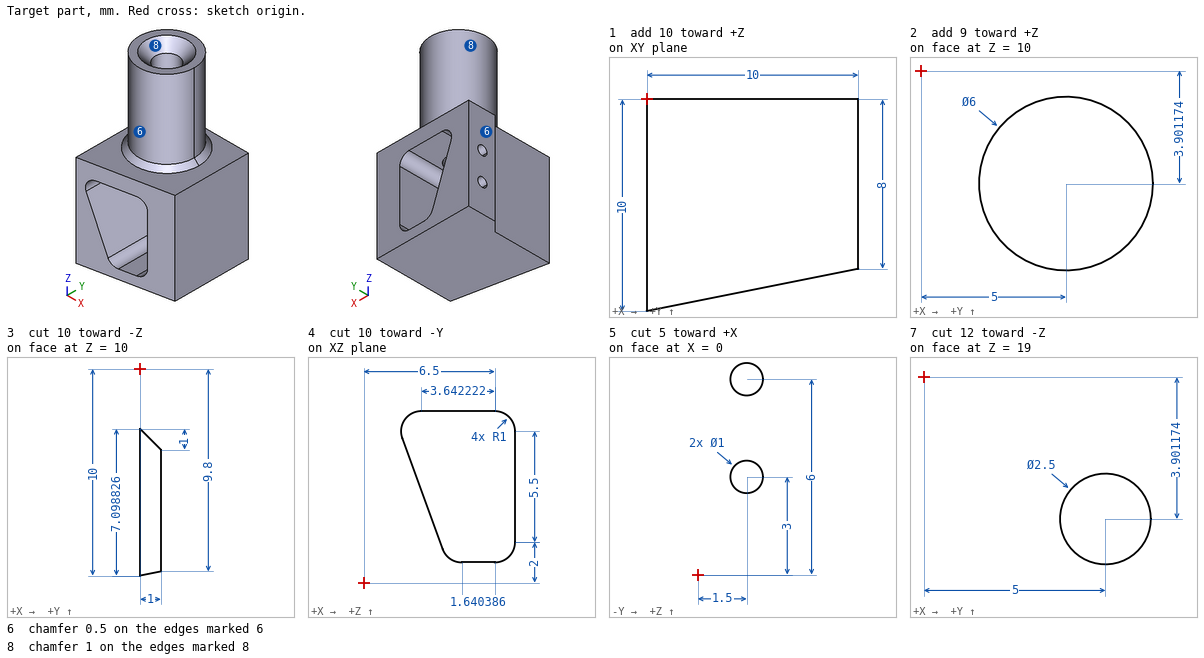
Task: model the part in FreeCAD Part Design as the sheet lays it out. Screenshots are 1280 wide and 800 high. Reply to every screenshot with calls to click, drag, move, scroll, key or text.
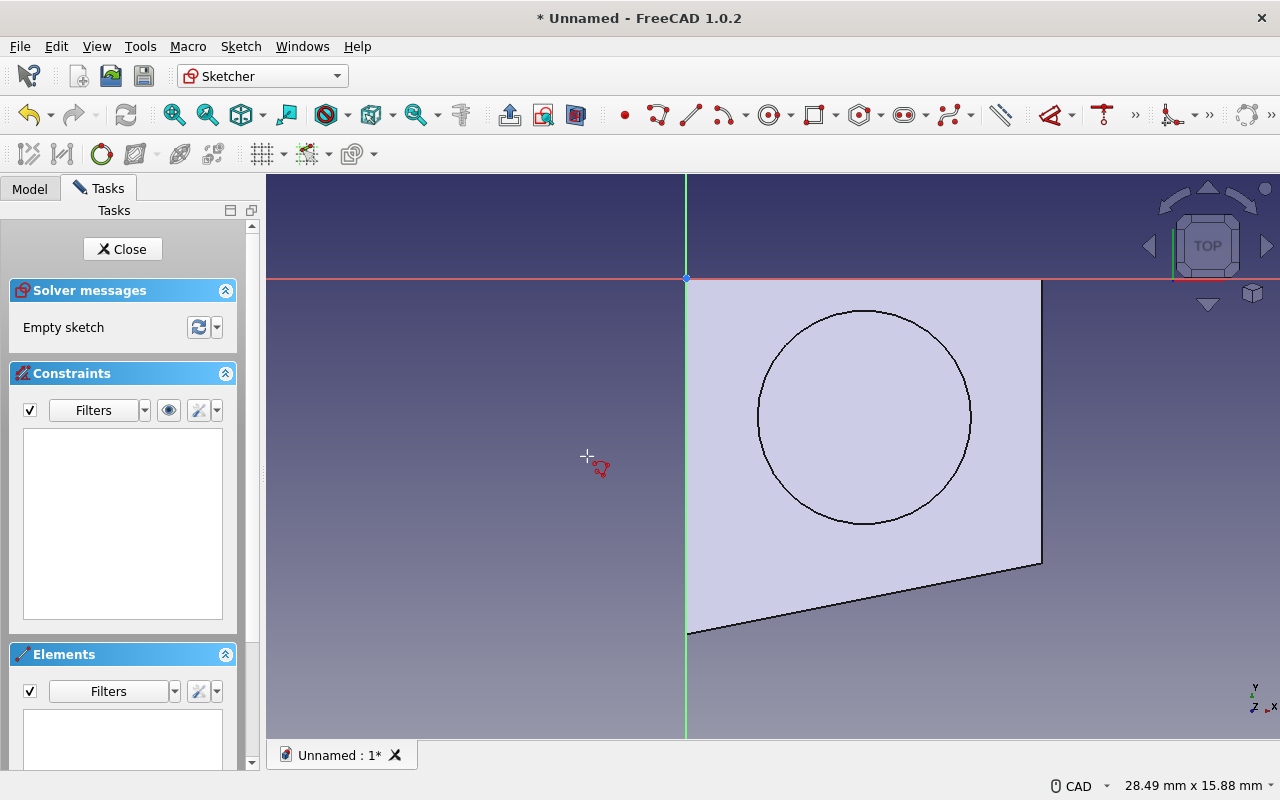
click(686, 382)
click(695, 634)
click(722, 627)
click(722, 417)
click(686, 383)
key(Escape)
key(Escape)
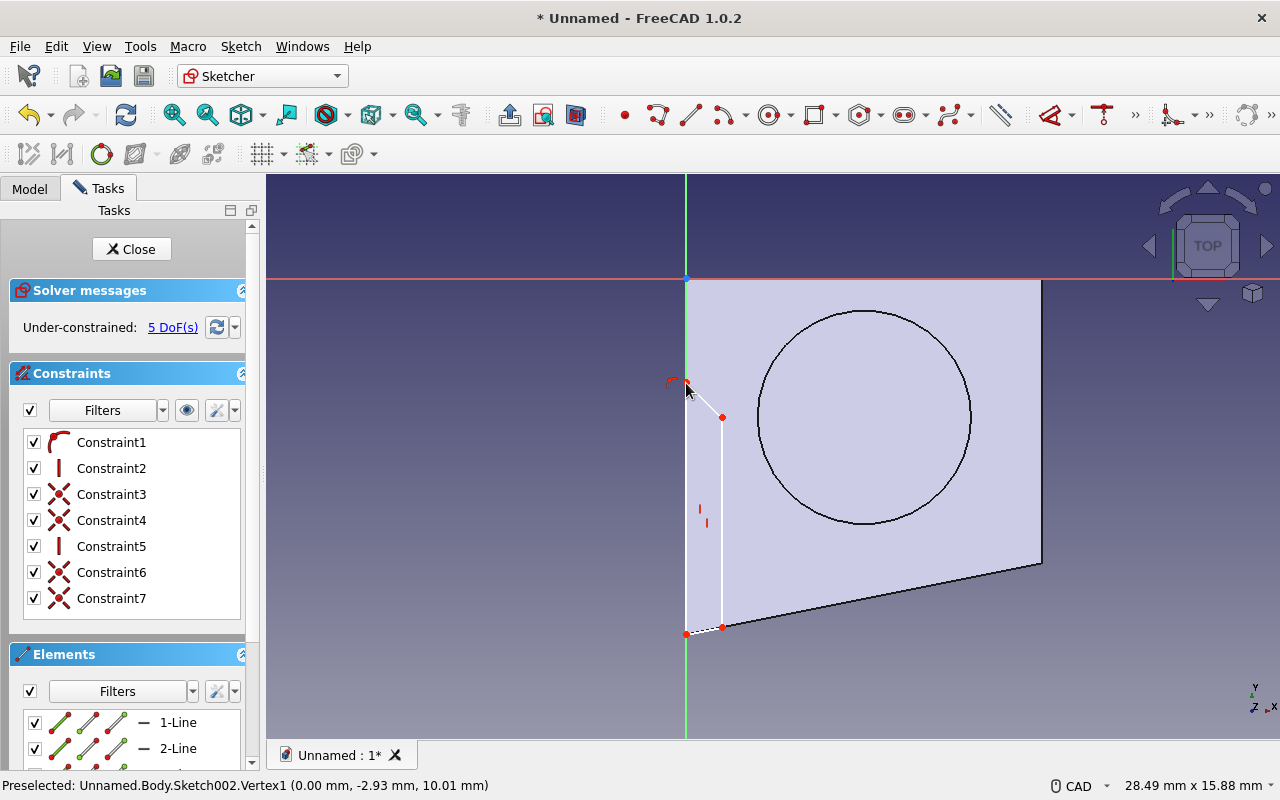
key(d)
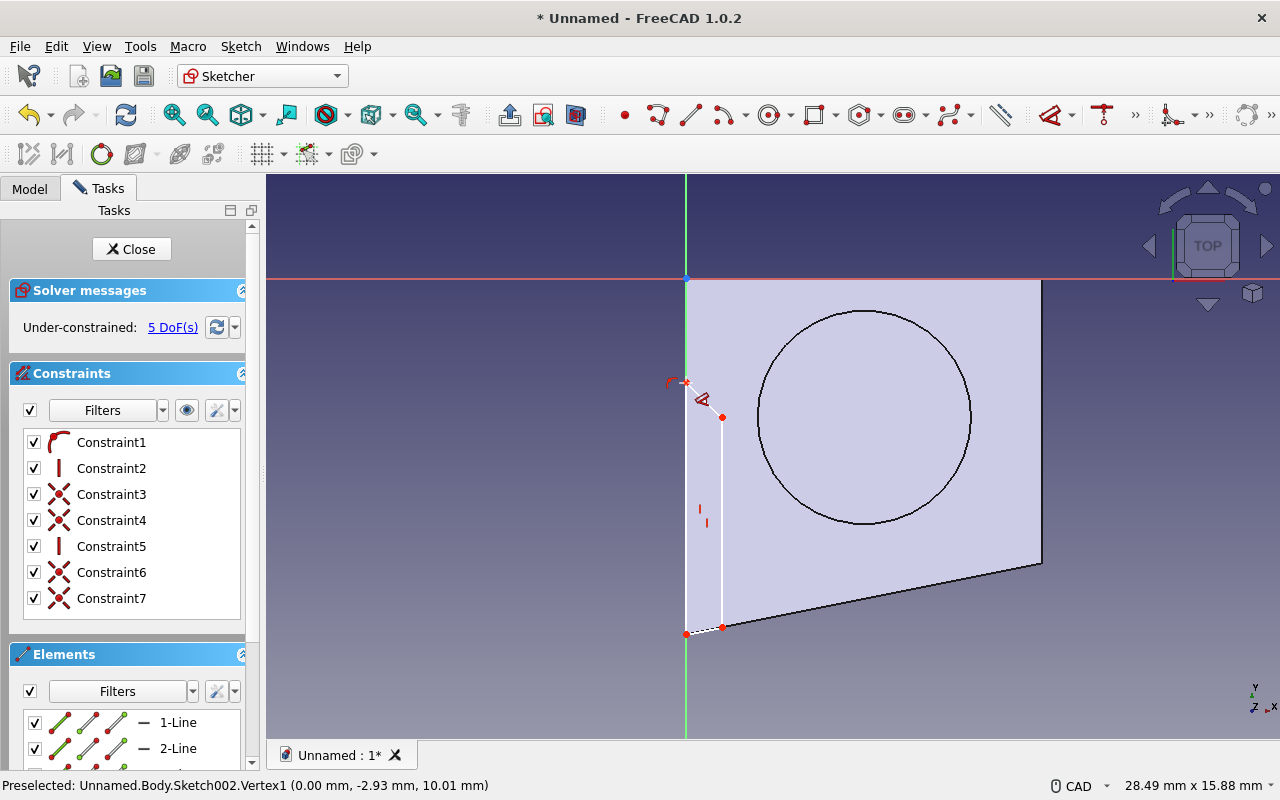
click(722, 628)
click(704, 245)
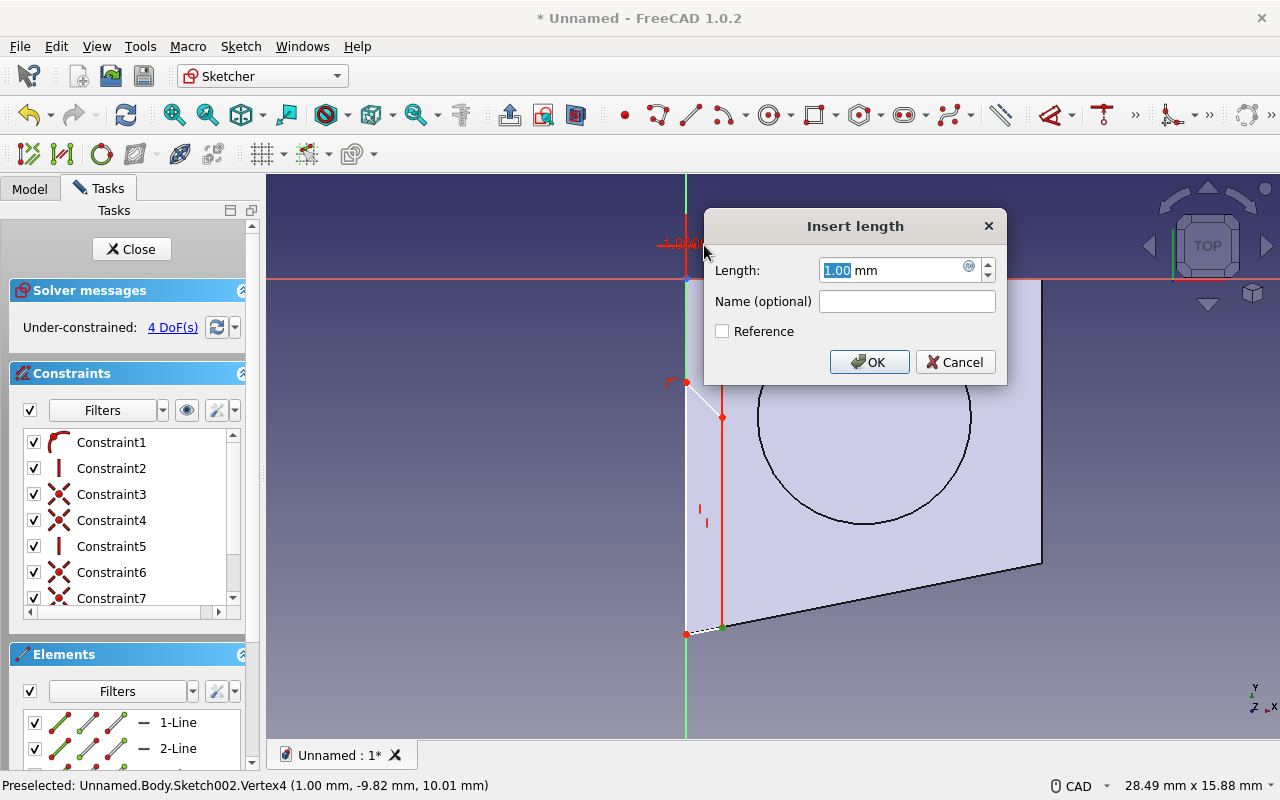
text(1)
key(Return)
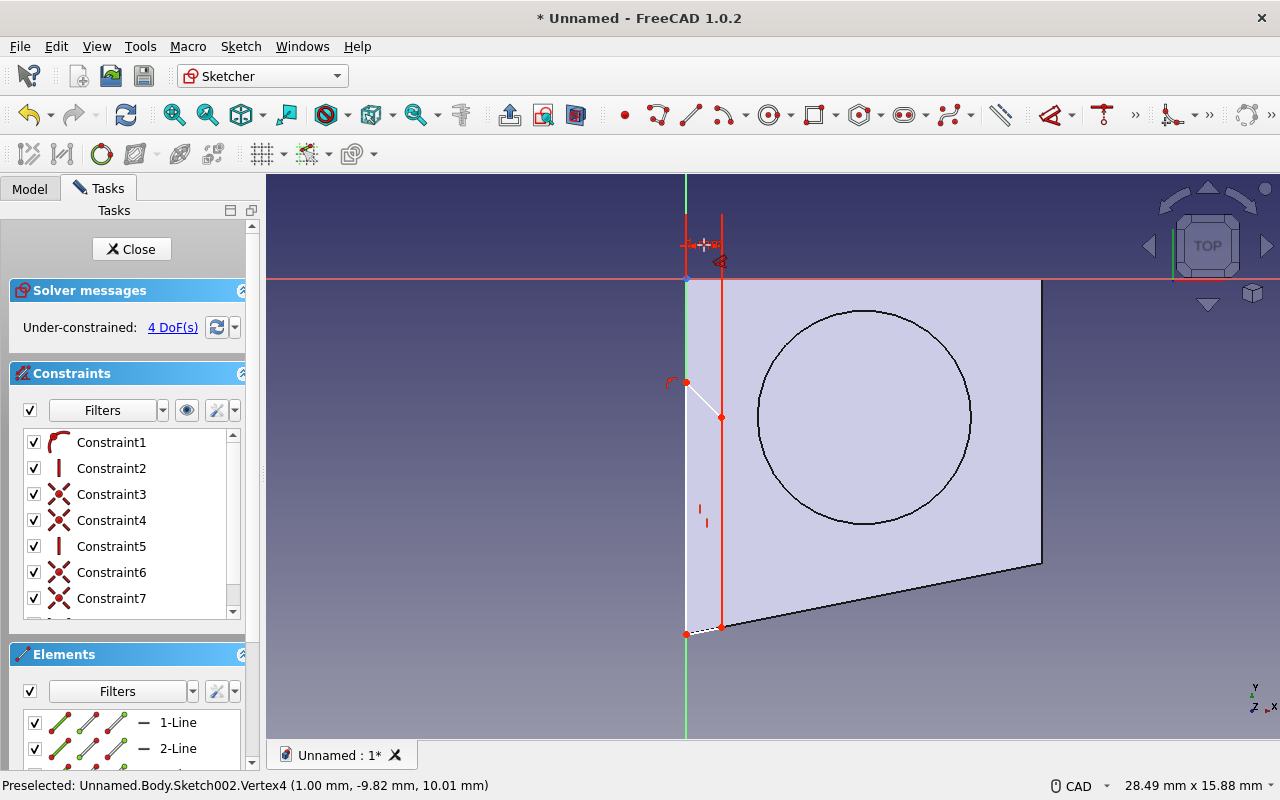
click(711, 408)
click(756, 401)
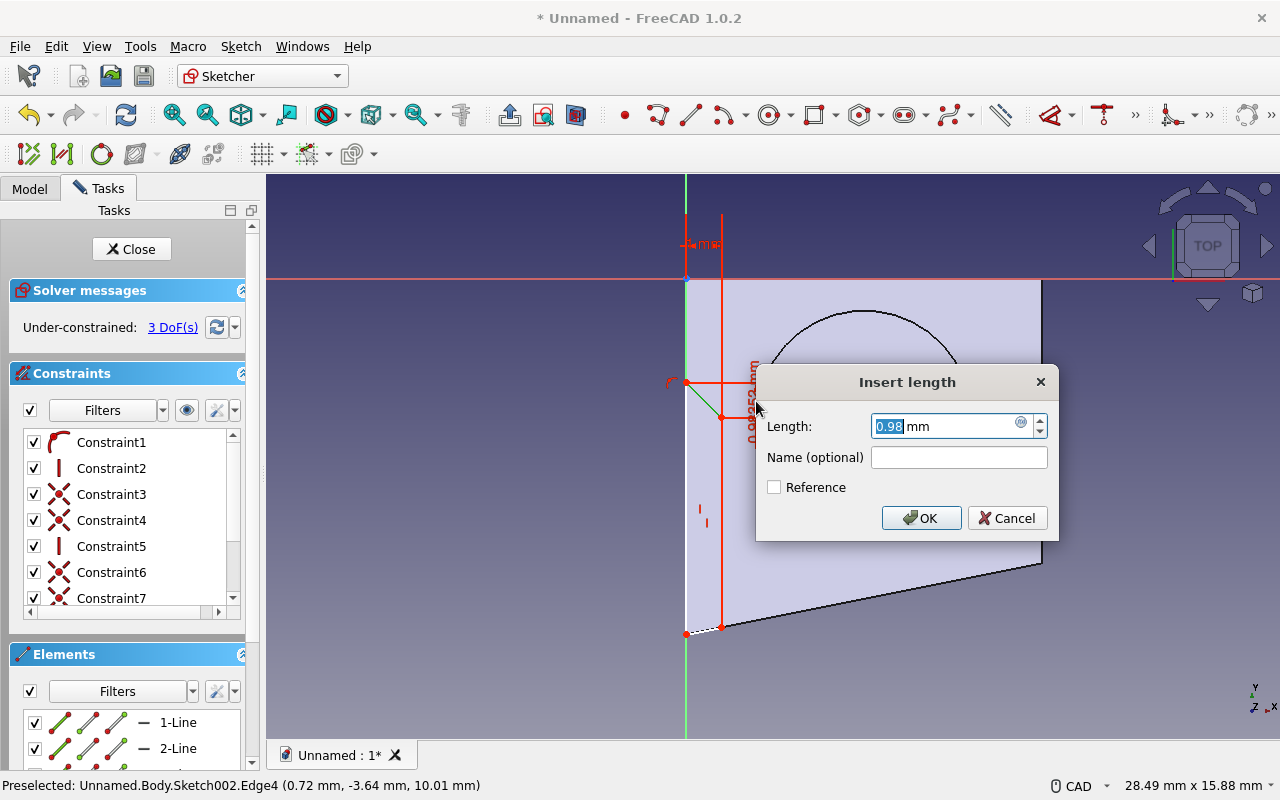
text(1)
key(Return)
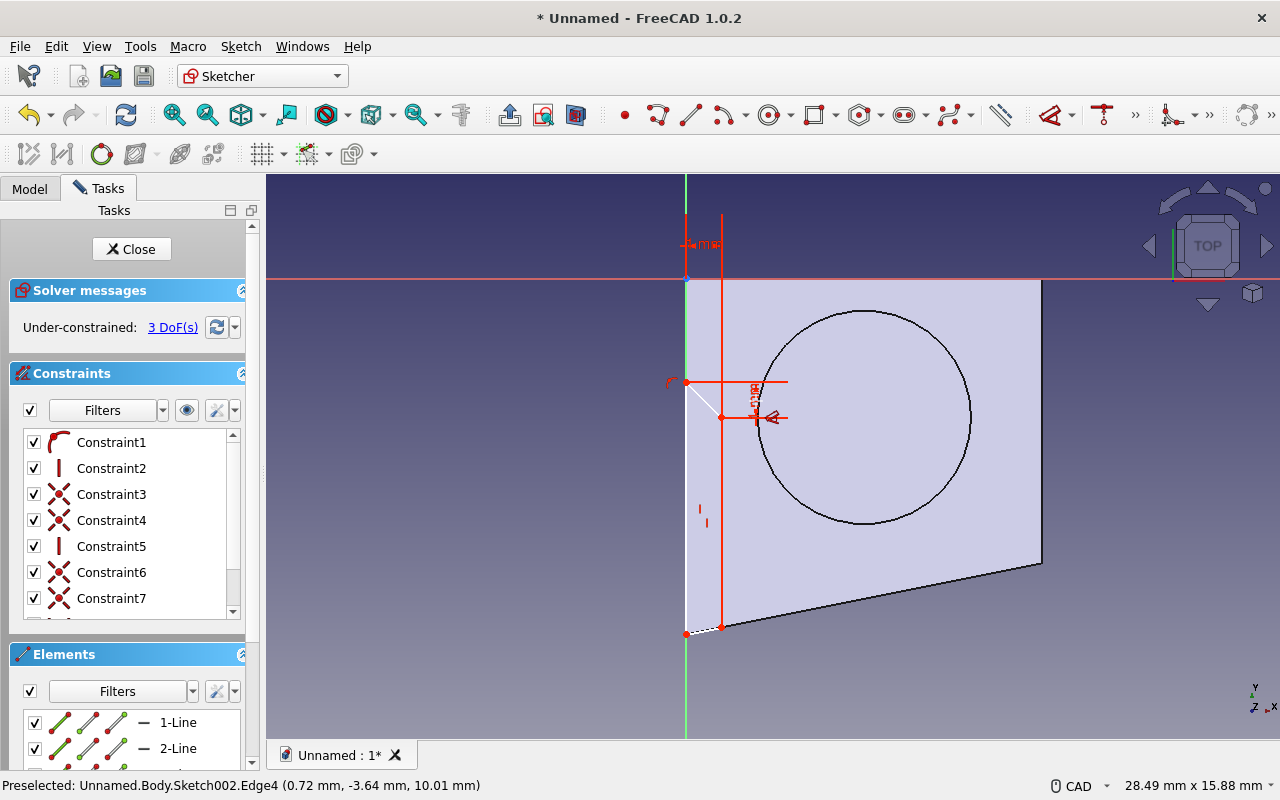
click(686, 635)
click(652, 457)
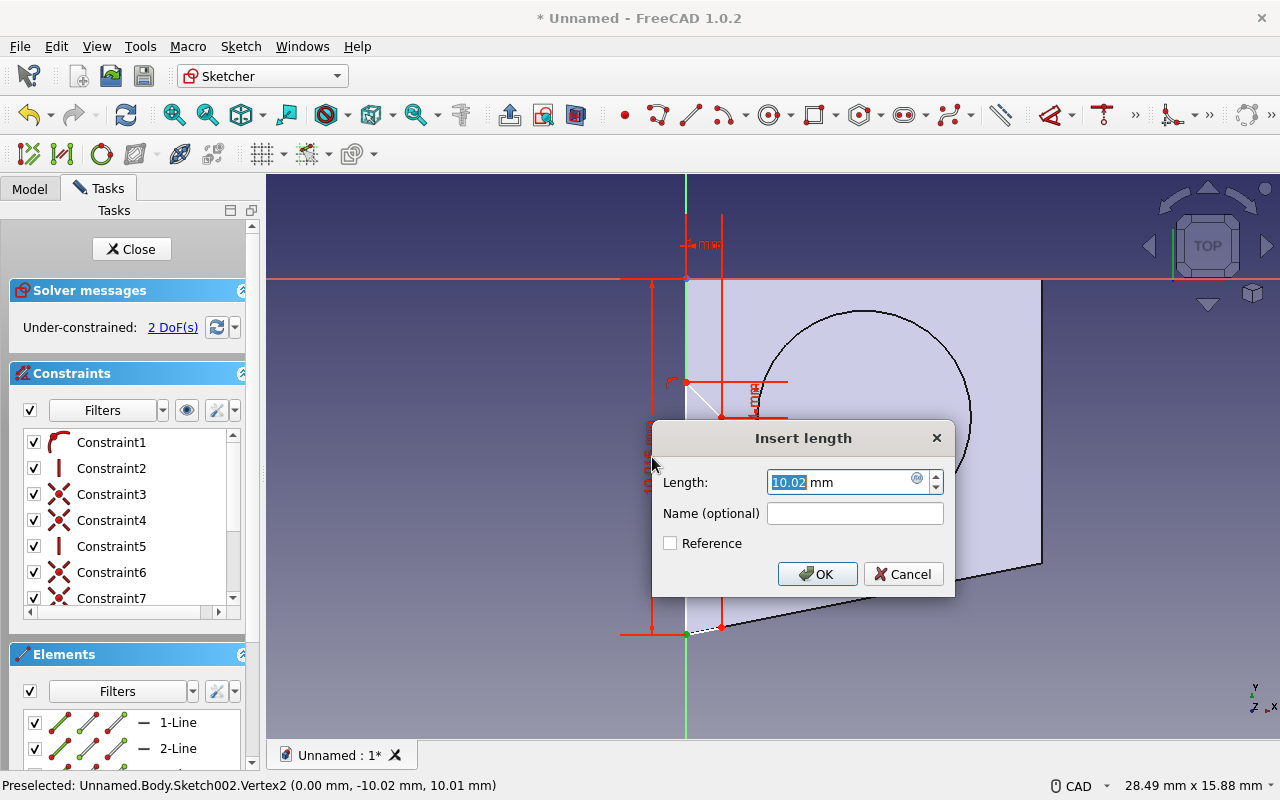
text(10)
key(Return)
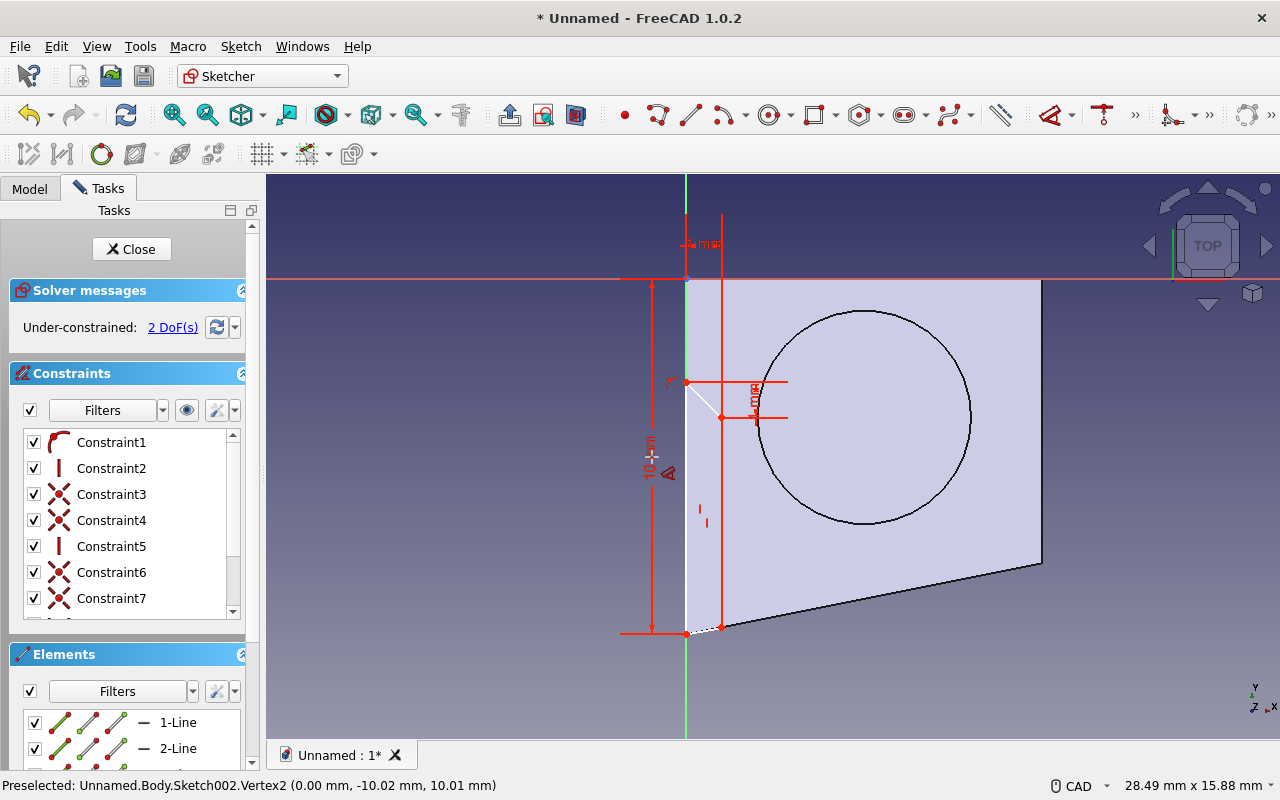
click(722, 628)
click(756, 453)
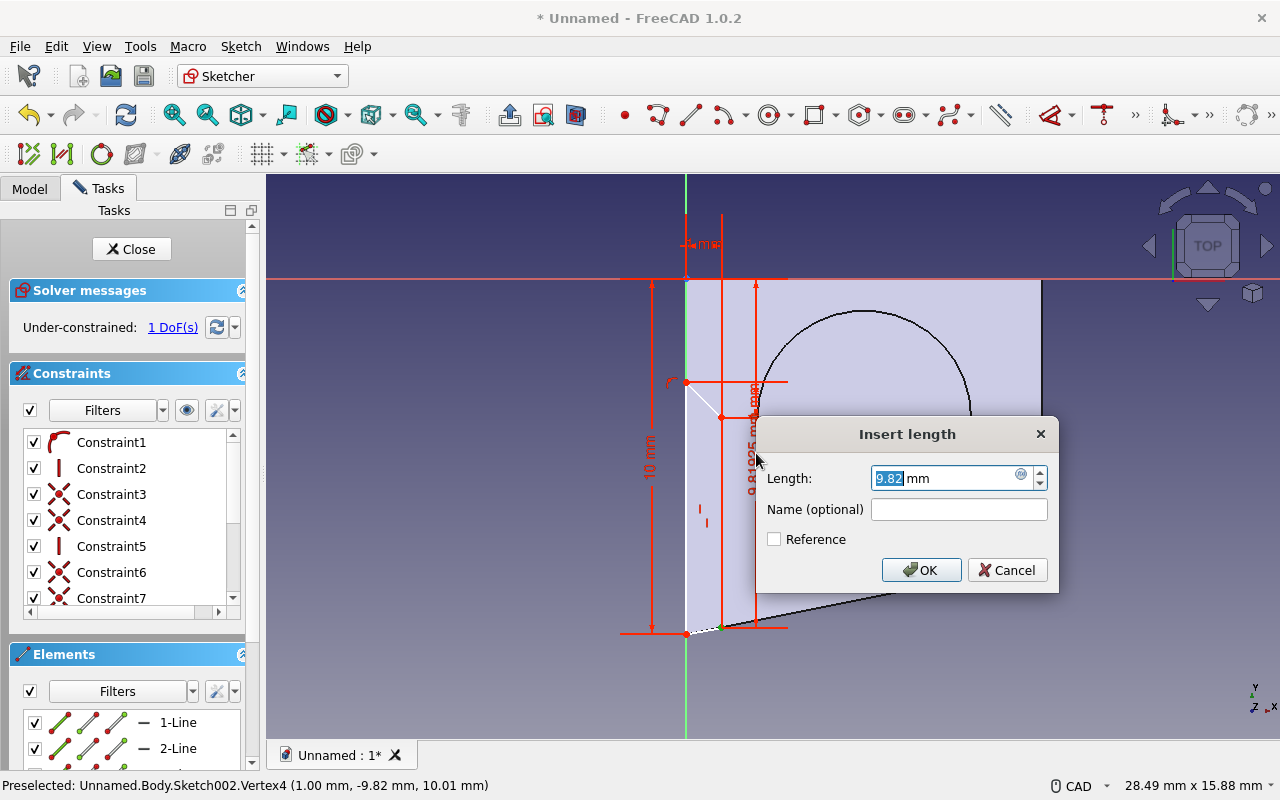
text(9.8)
key(Return)